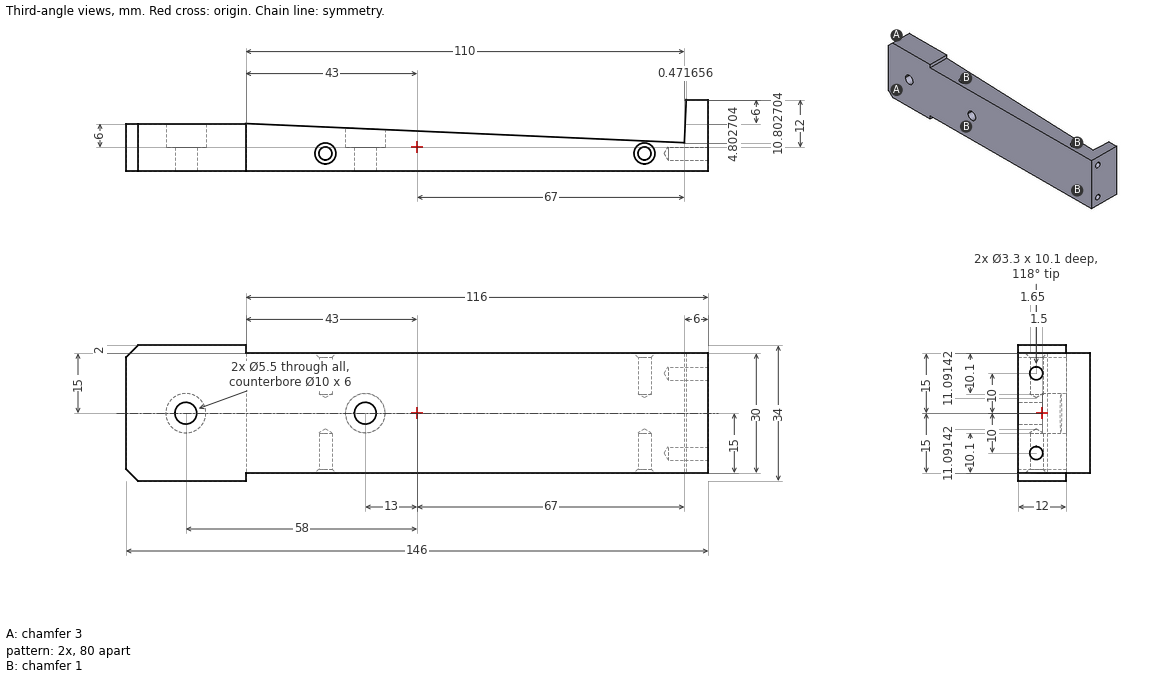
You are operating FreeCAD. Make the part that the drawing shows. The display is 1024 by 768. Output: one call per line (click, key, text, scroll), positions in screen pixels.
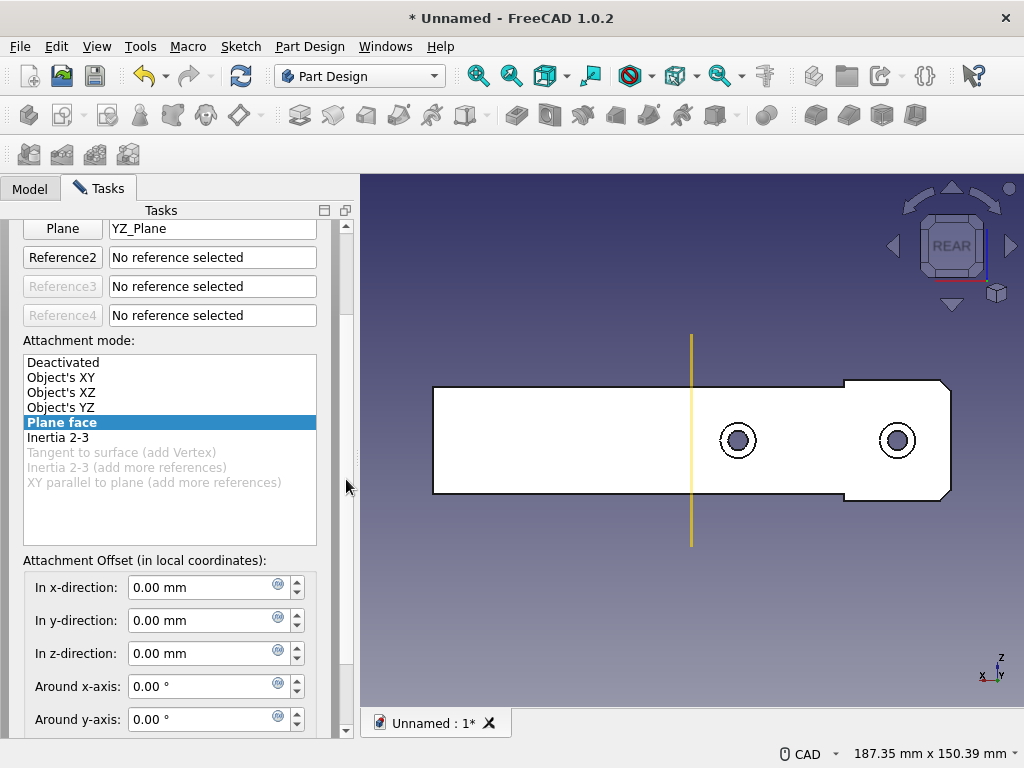
triple_click(210, 654)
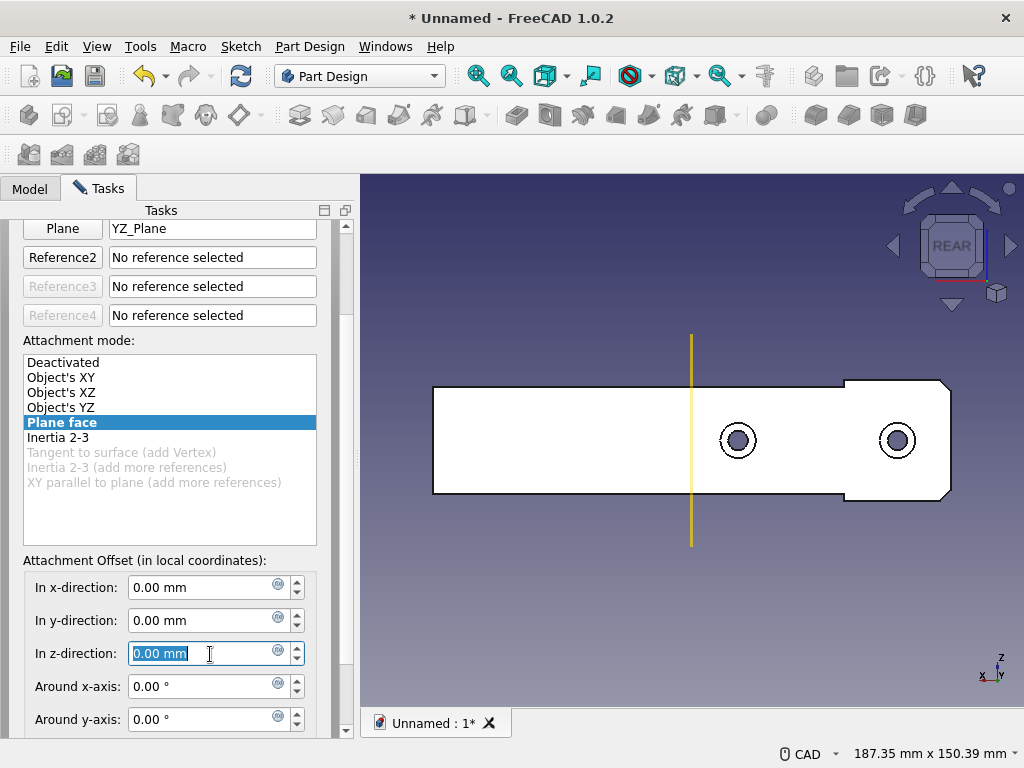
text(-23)
key(Tab)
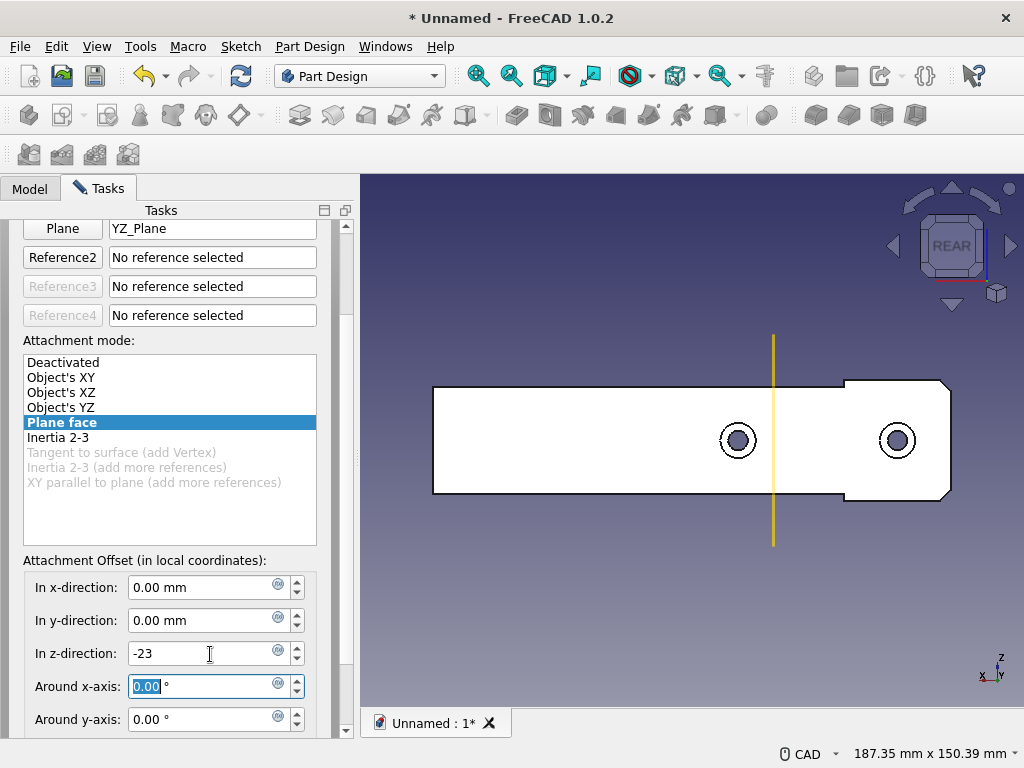
scroll(346, 479, up, 3)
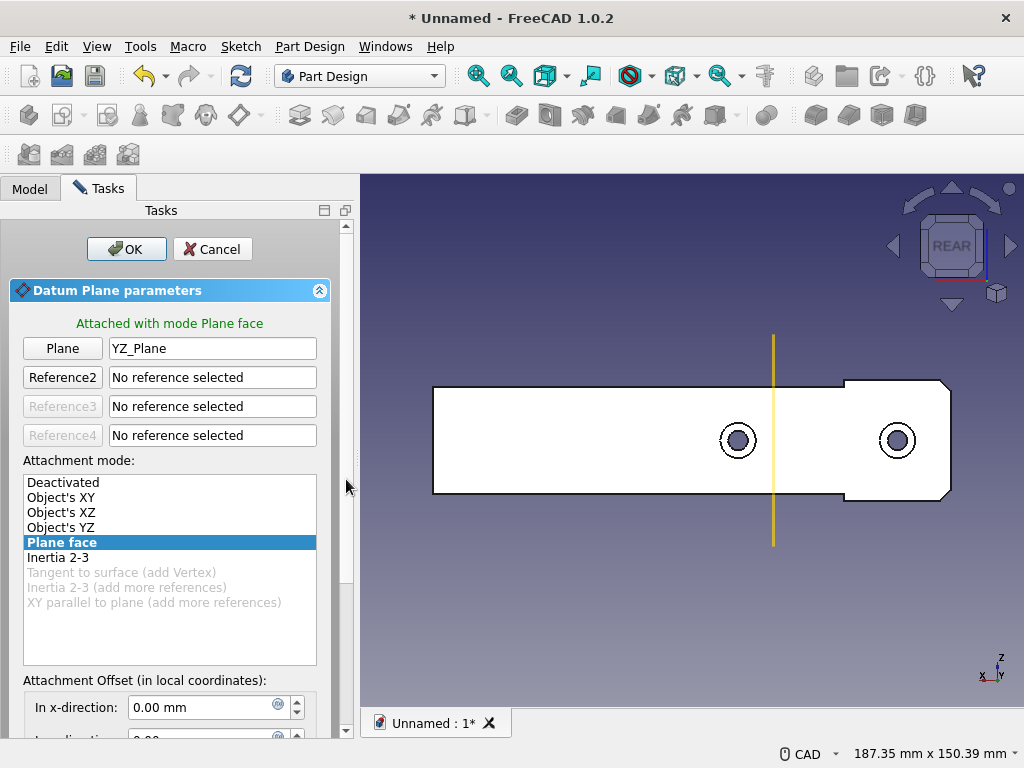
click(127, 249)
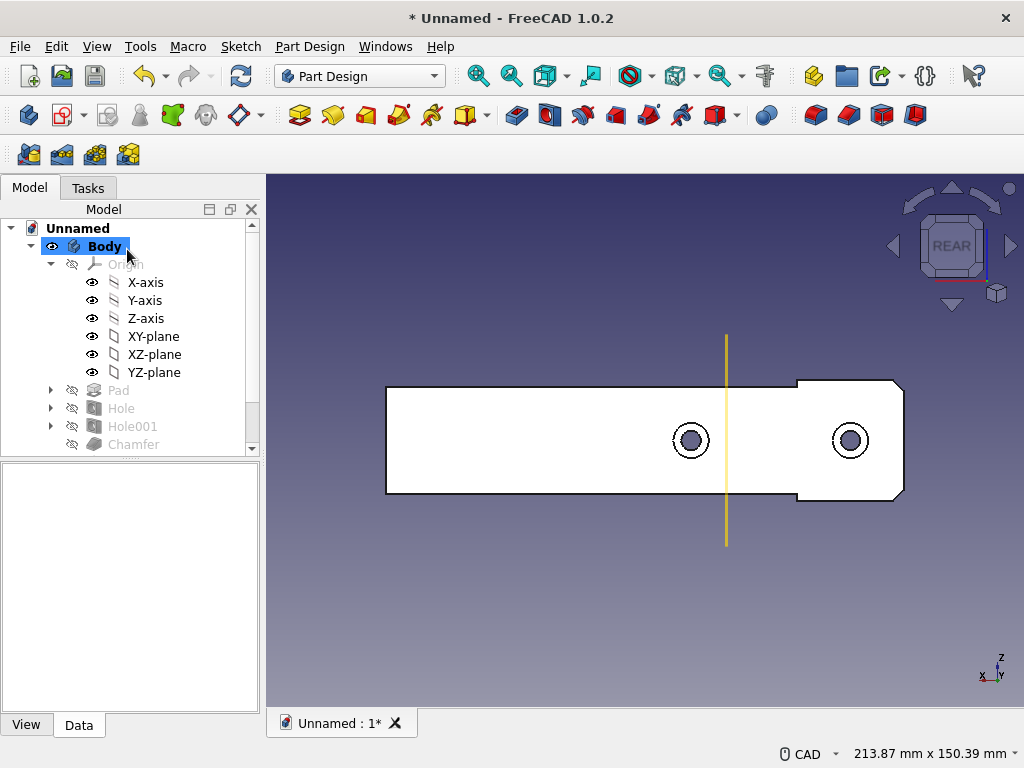
scroll(101, 332, down, 3)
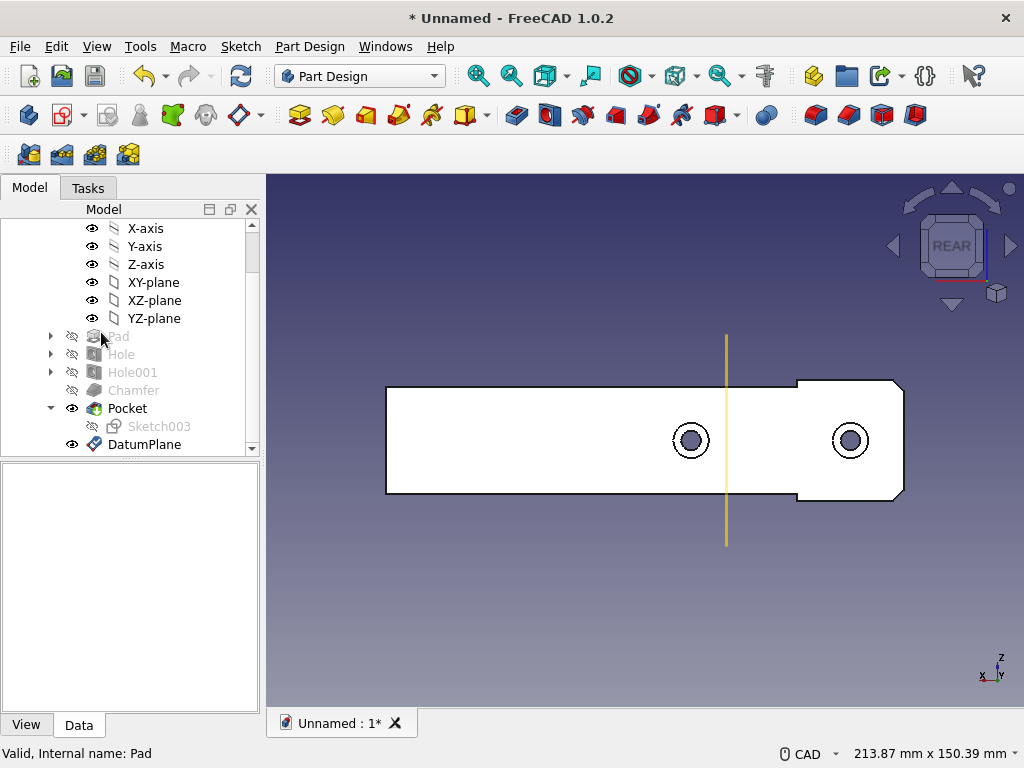
click(117, 444)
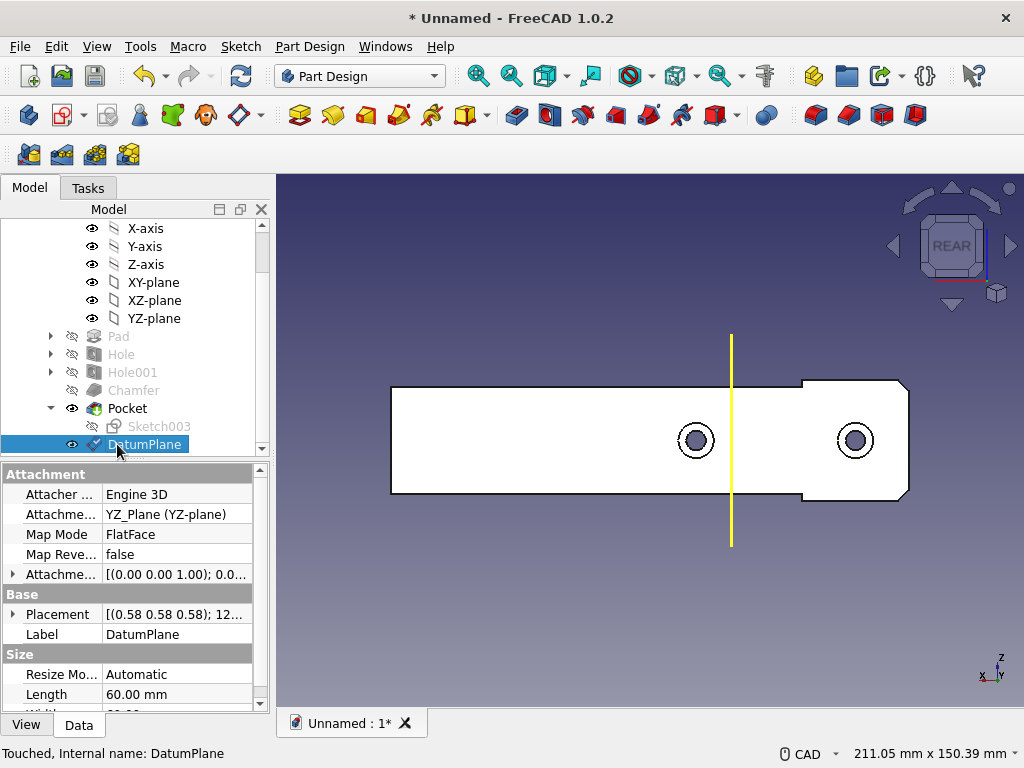
click(62, 116)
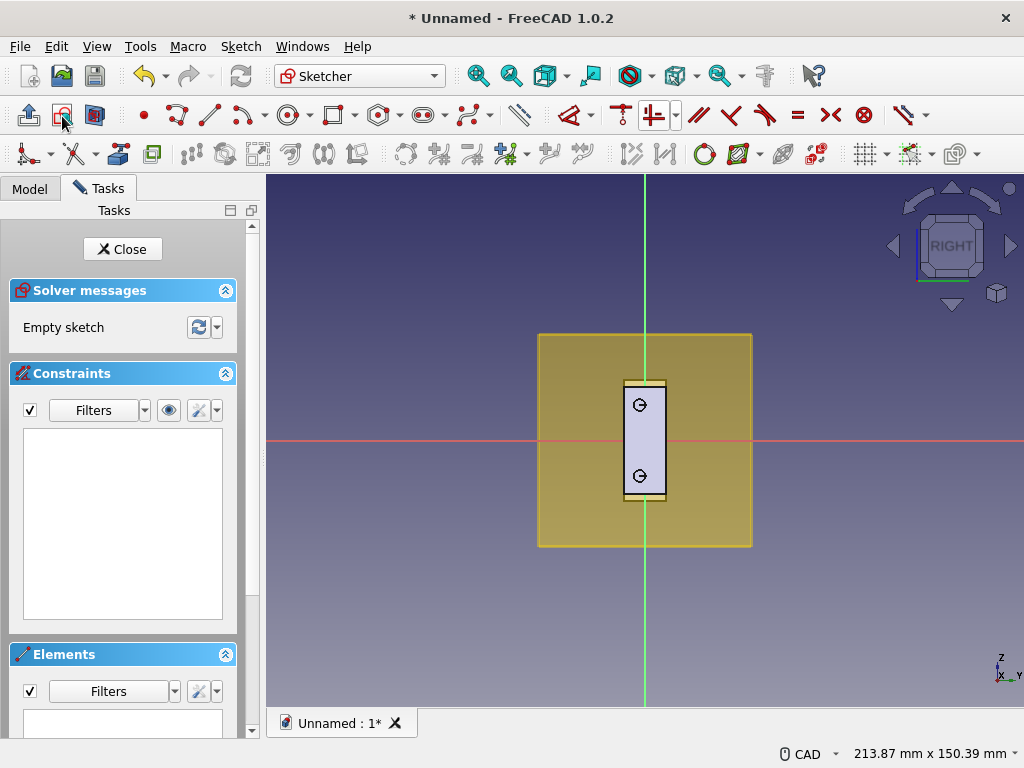
click(95, 116)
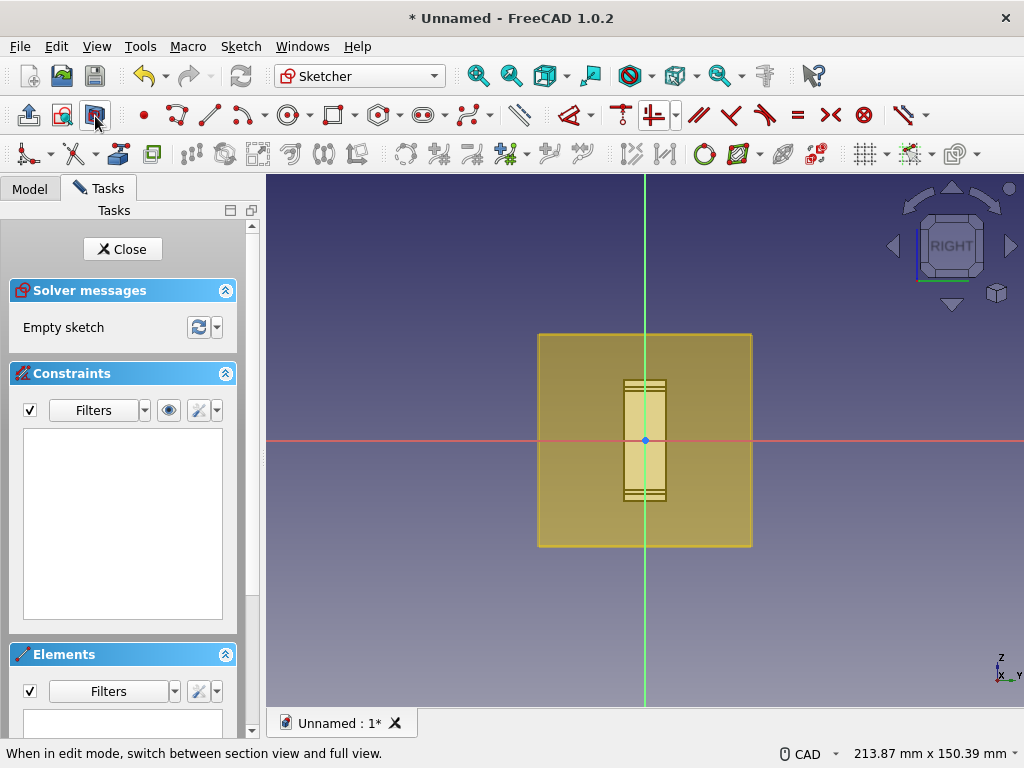
scroll(652, 410, up, 9)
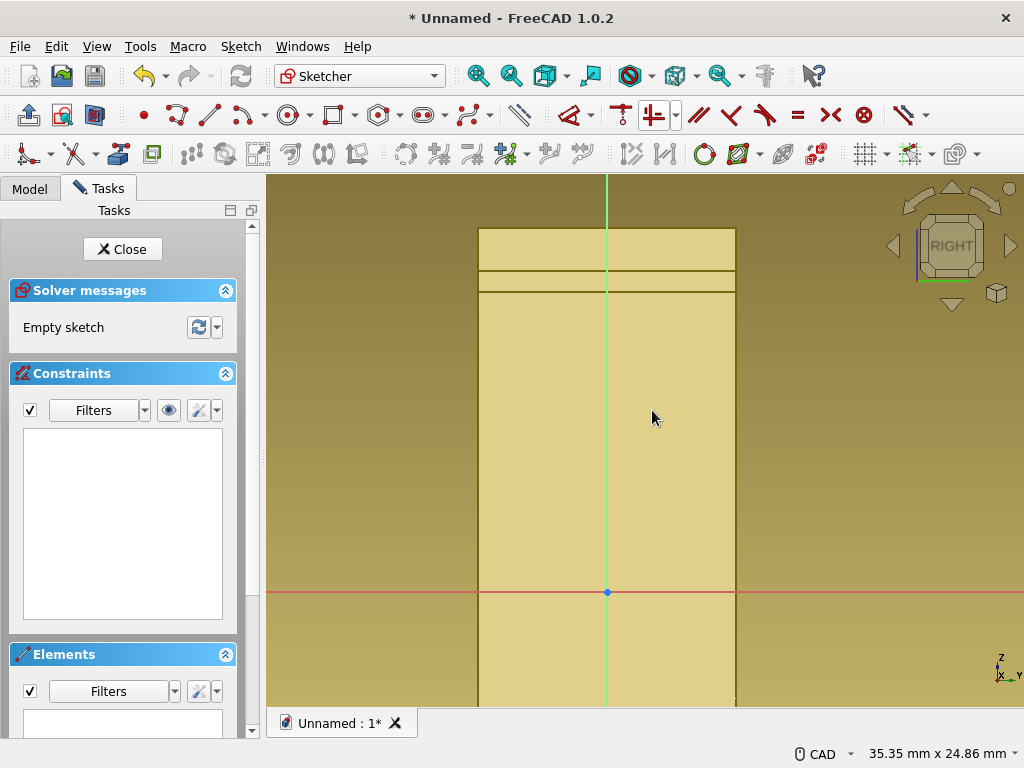
click(177, 116)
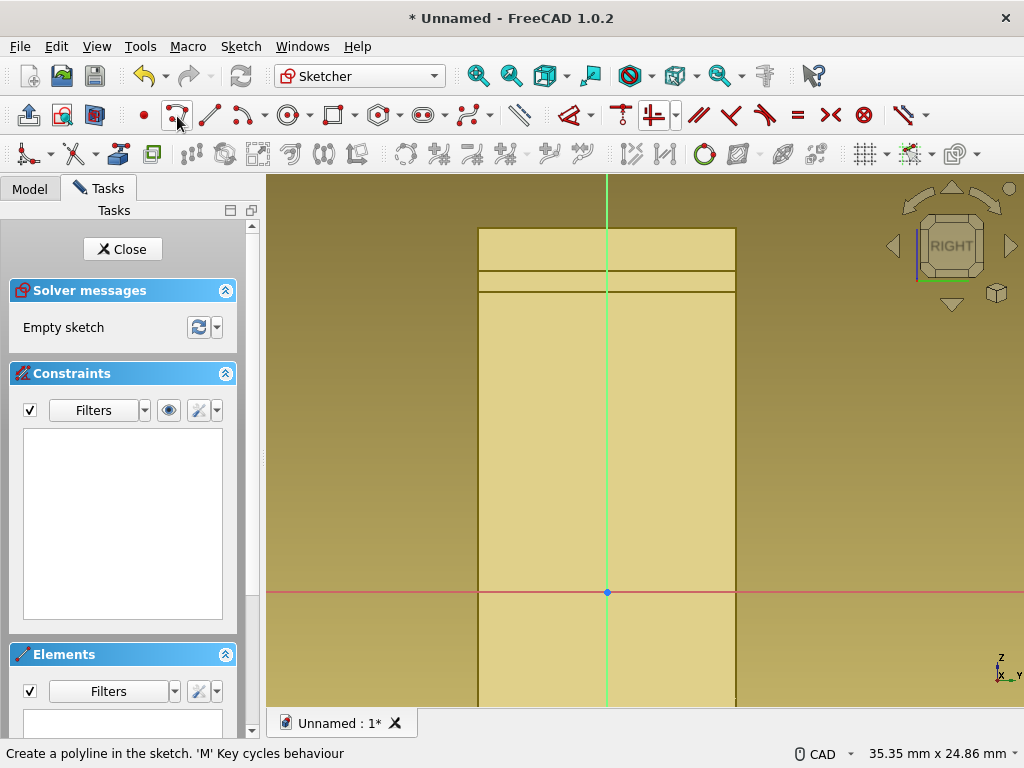
click(575, 508)
click(575, 271)
click(540, 271)
click(540, 487)
click(575, 509)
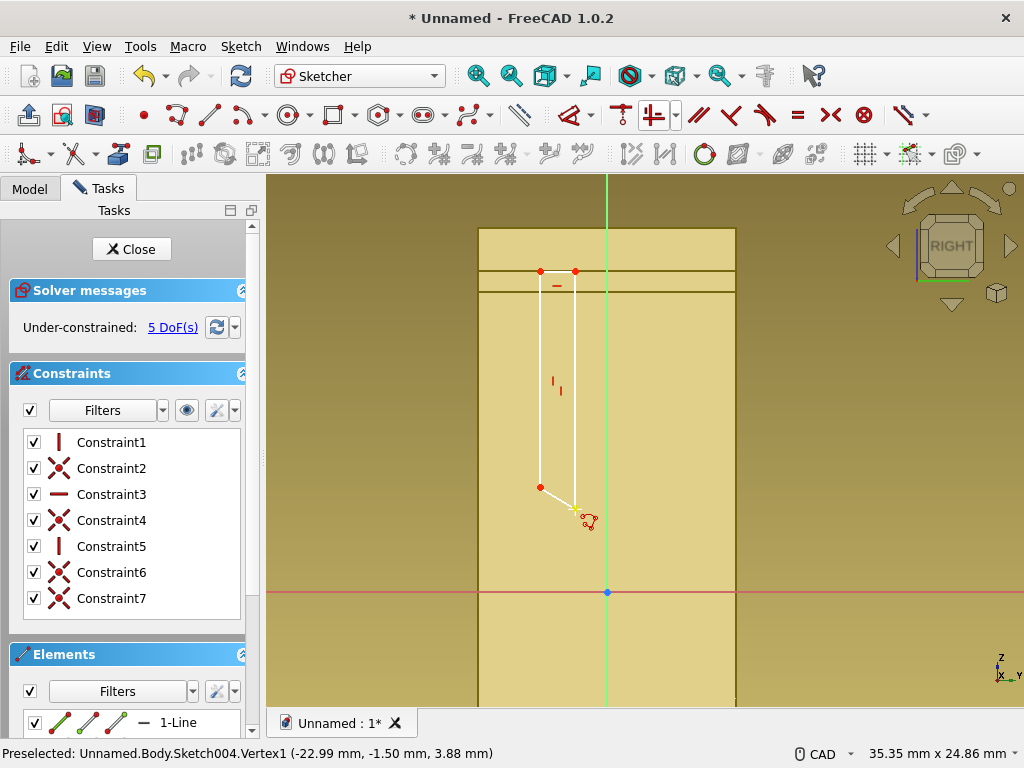
click(210, 116)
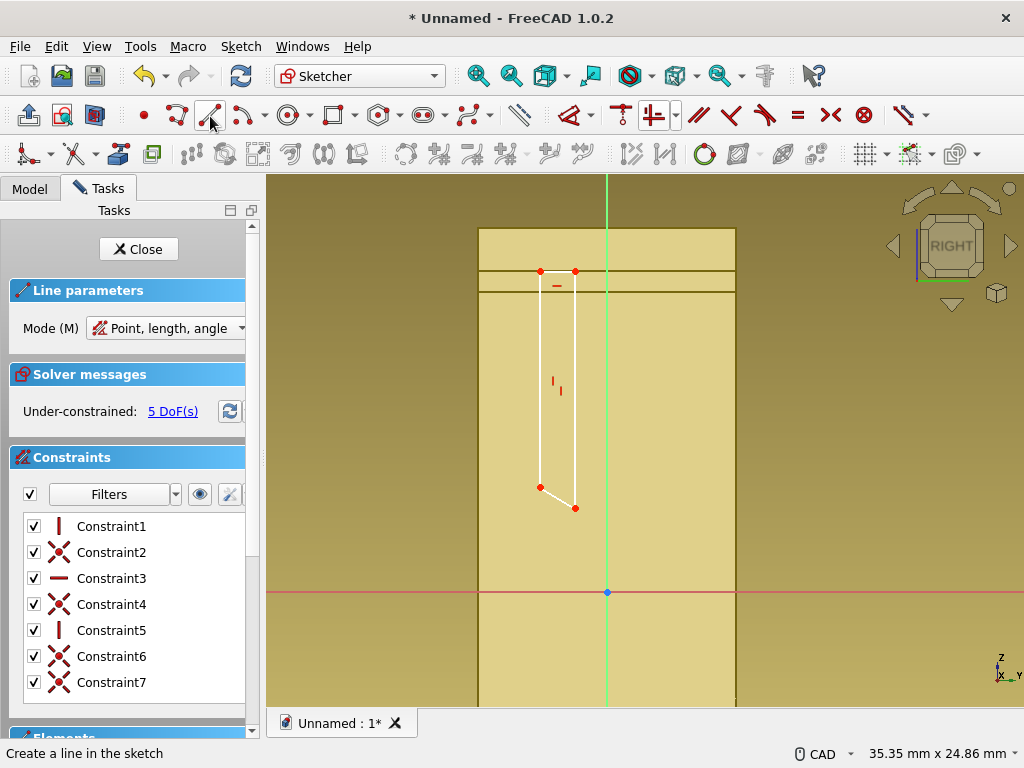
click(575, 532)